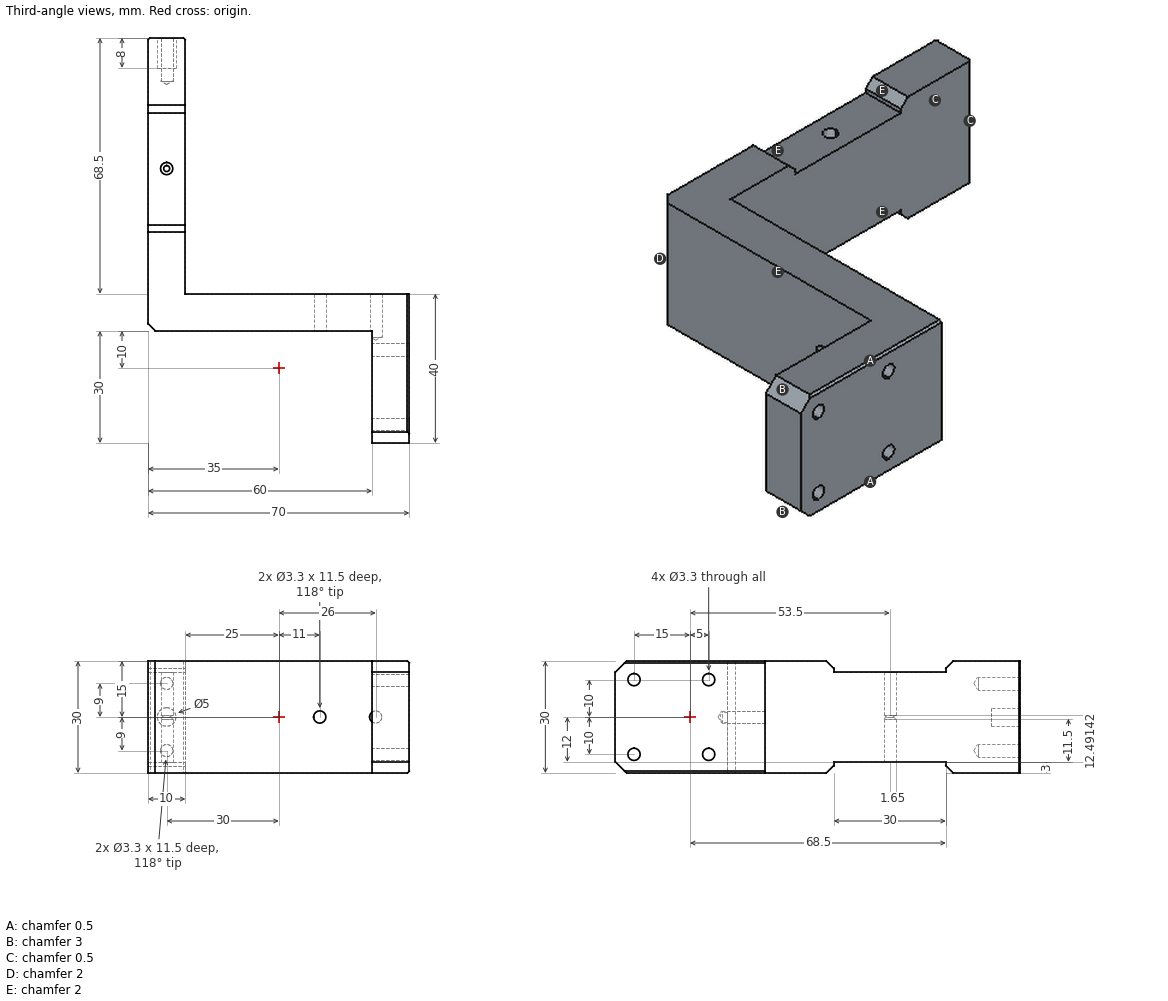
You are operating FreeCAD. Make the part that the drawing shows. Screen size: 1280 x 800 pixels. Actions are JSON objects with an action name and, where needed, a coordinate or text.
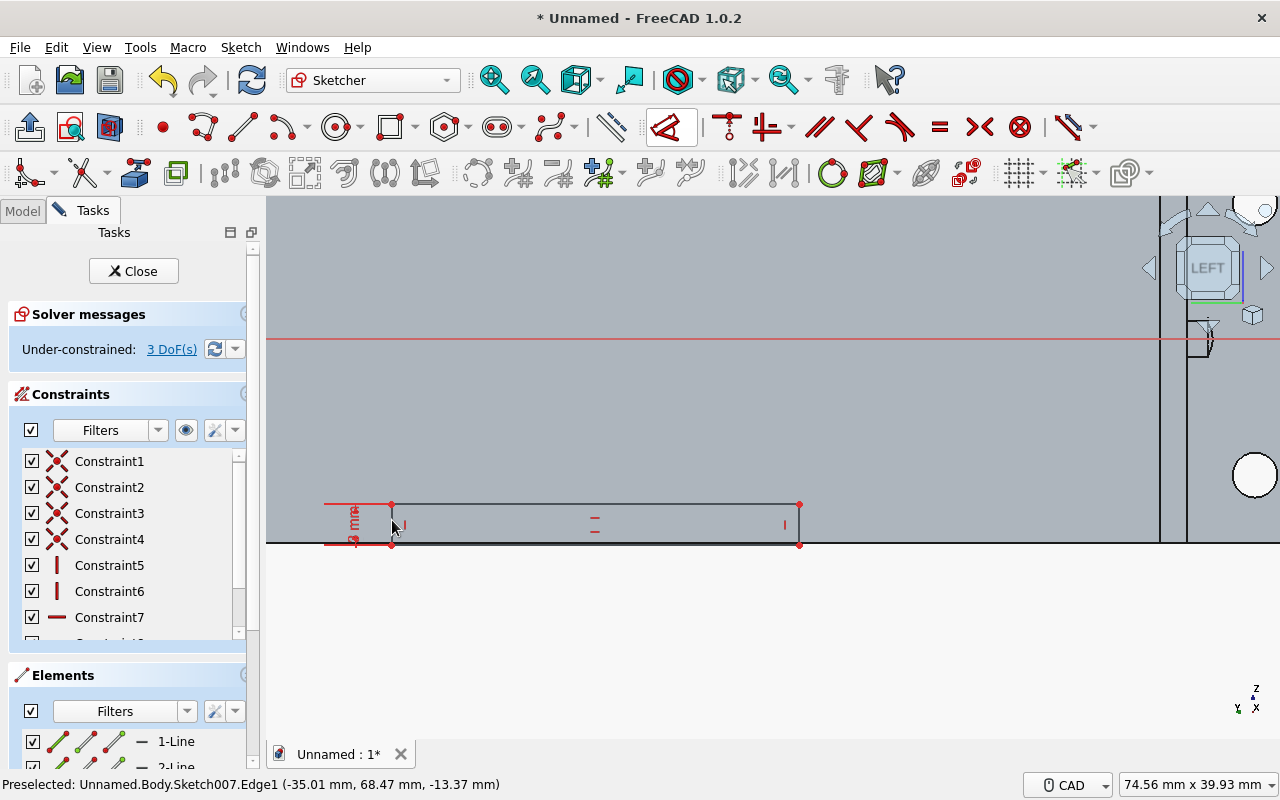
{"action": "left_click", "coordinate": [514, 545]}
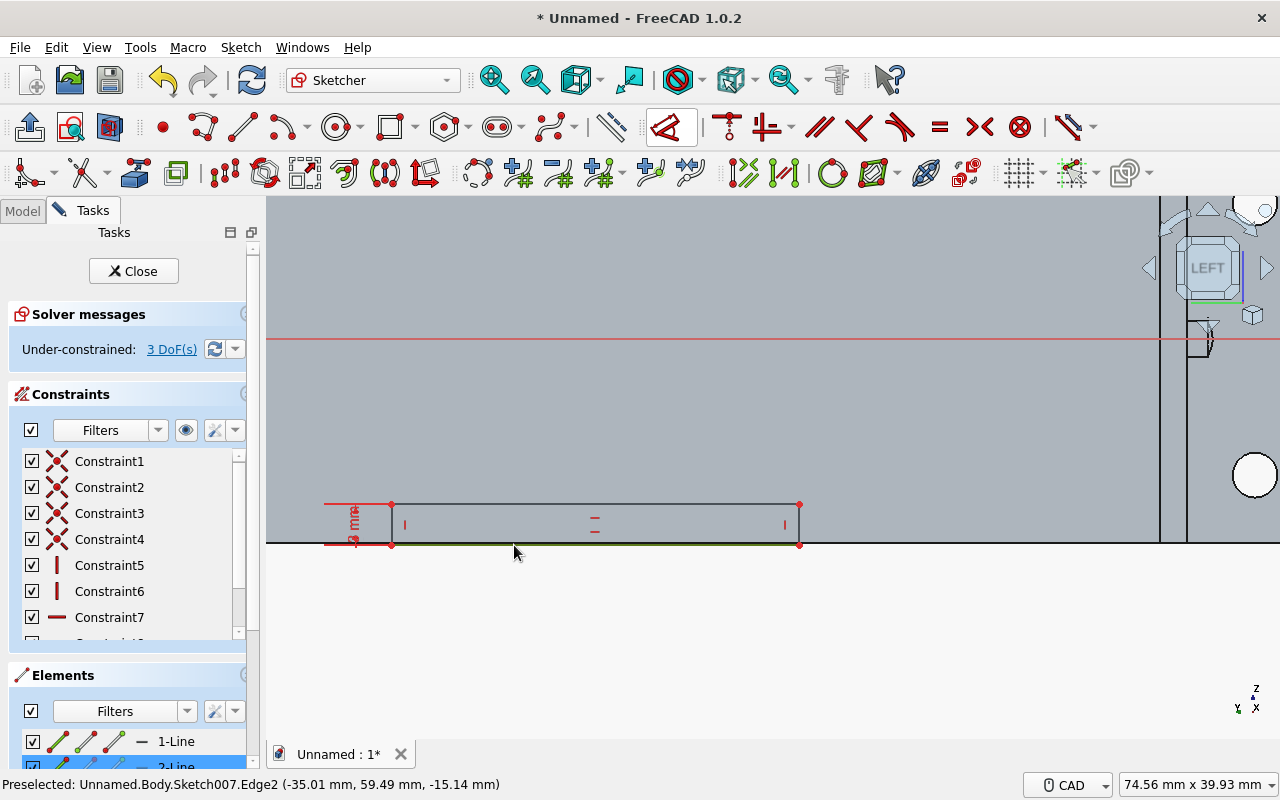
{"action": "key", "text": "l"}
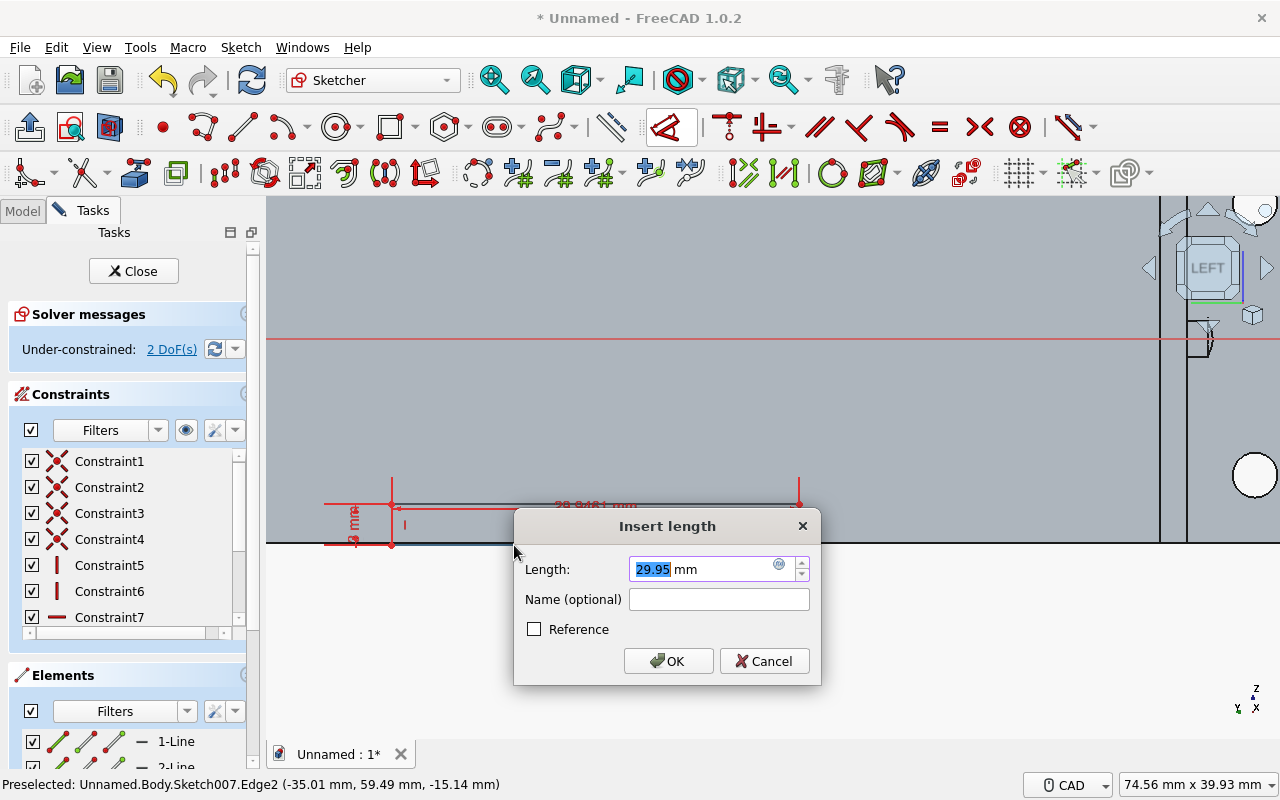
{"action": "type", "text": "30"}
{"action": "key", "text": "Return"}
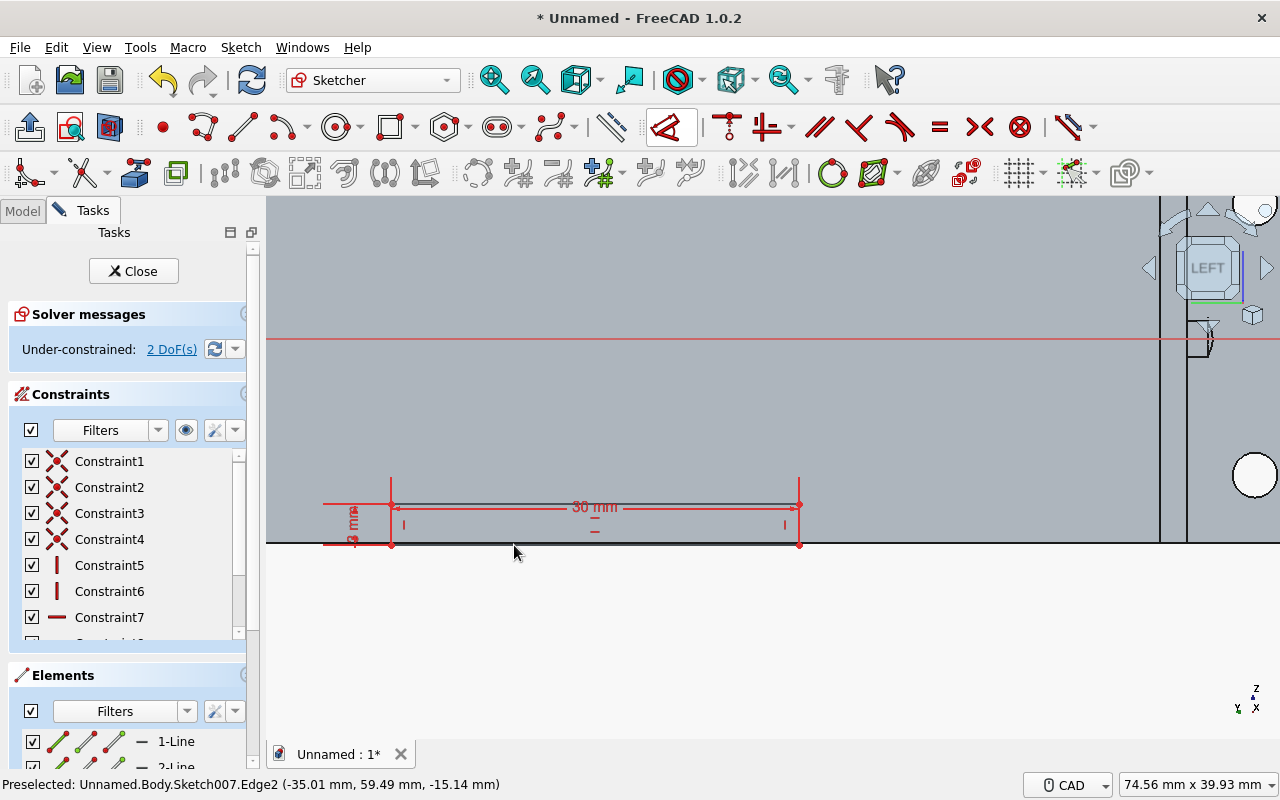
{"action": "left_click", "coordinate": [391, 504]}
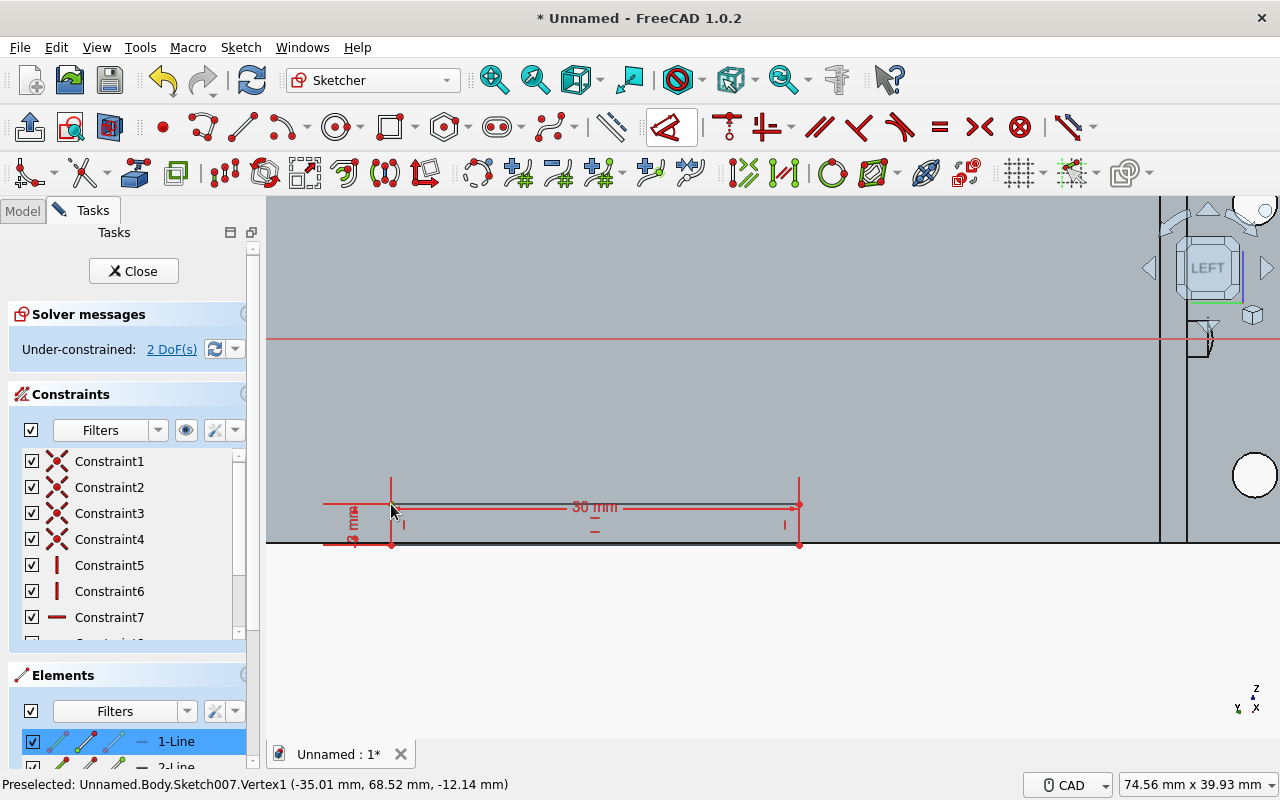
{"action": "left_click", "coordinate": [692, 128]}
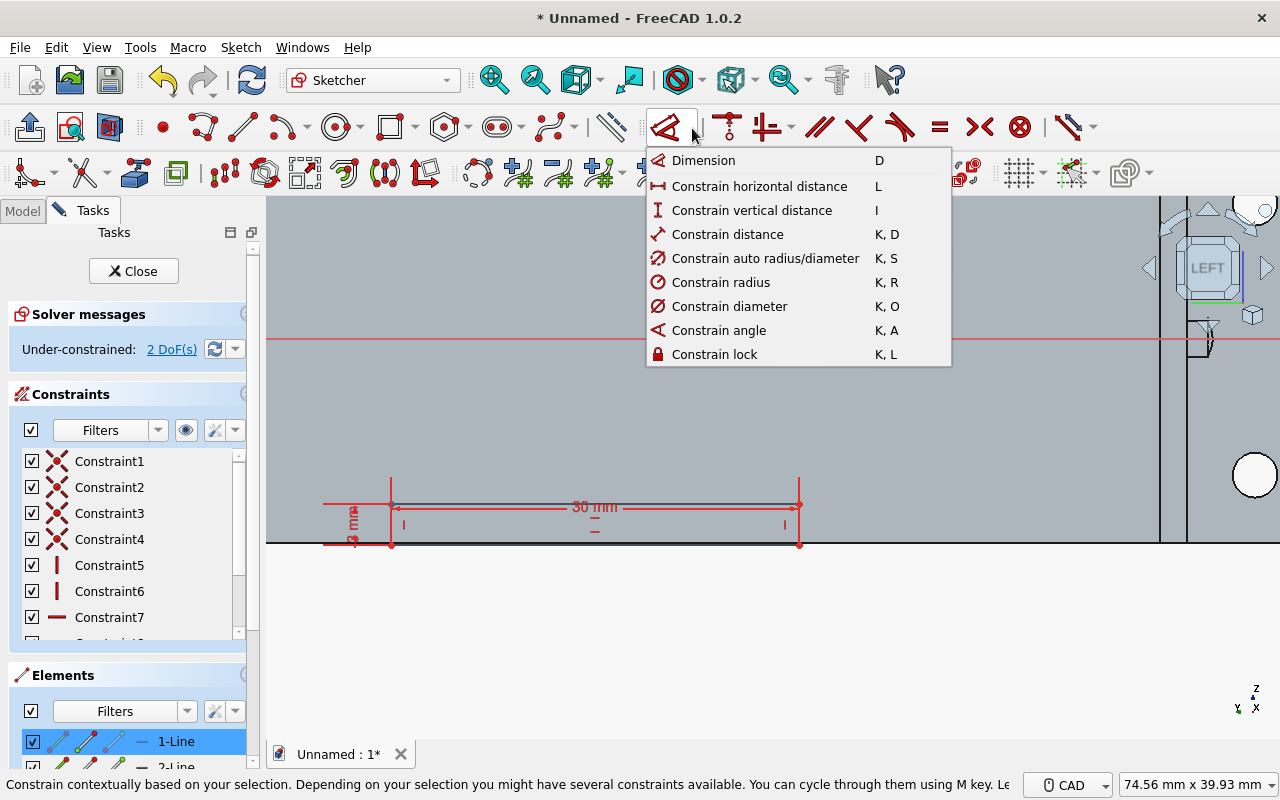
{"action": "left_click", "coordinate": [799, 210]}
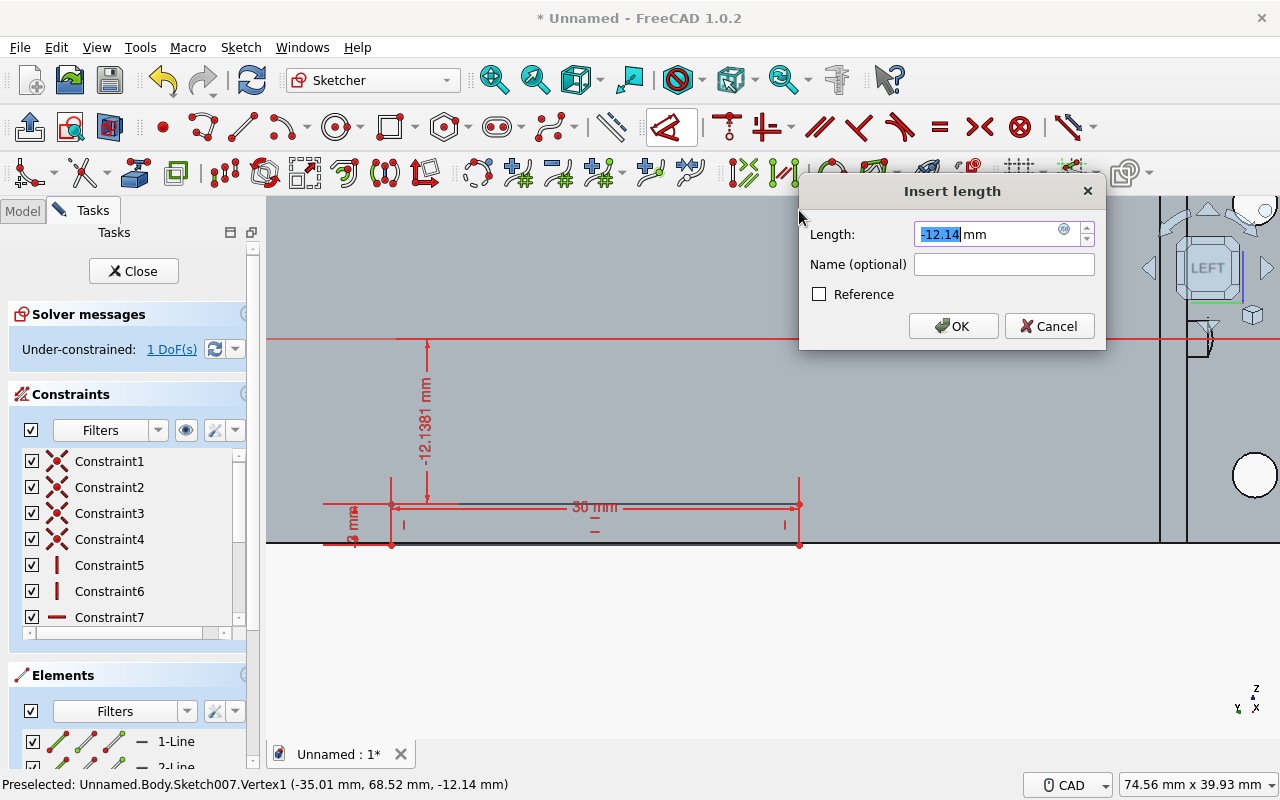
{"action": "type", "text": "-12"}
{"action": "key", "text": "Return"}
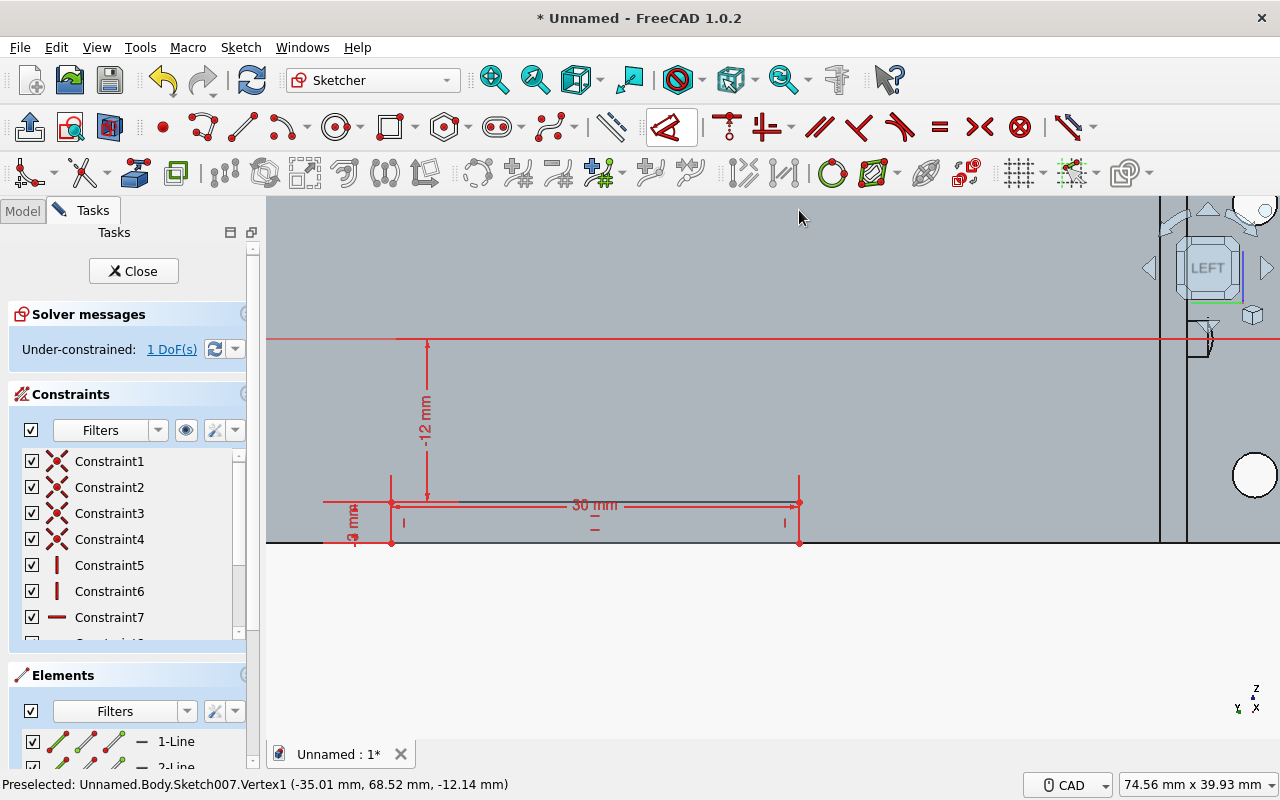
{"action": "left_click", "coordinate": [391, 502]}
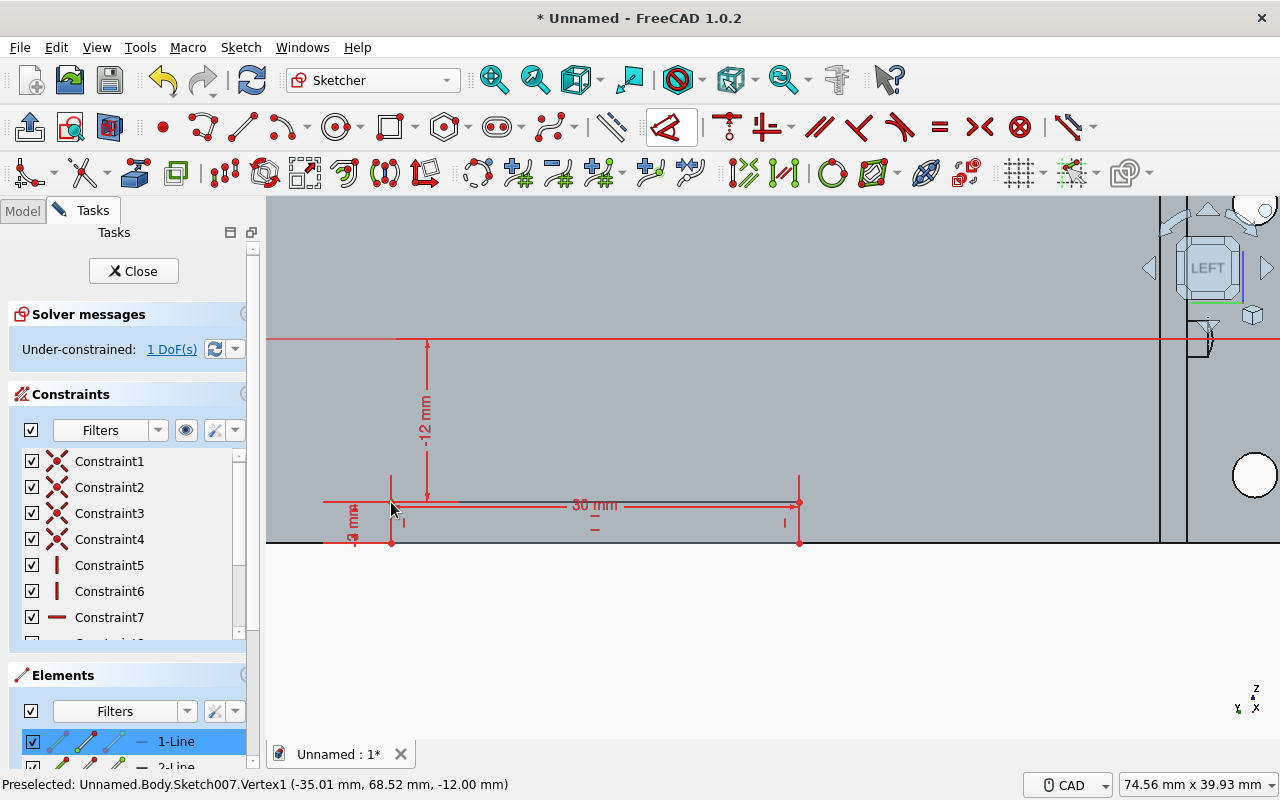
{"action": "left_click", "coordinate": [692, 128]}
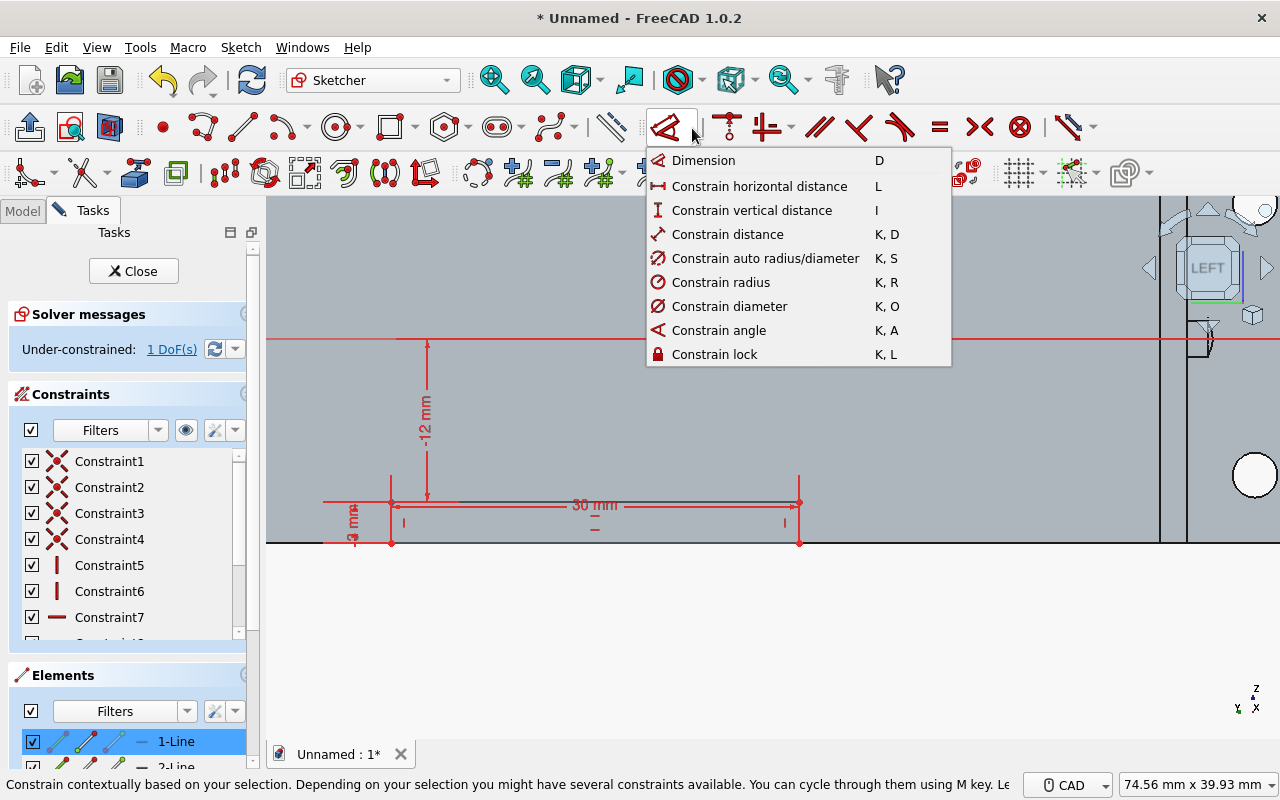
{"action": "left_click", "coordinate": [799, 186]}